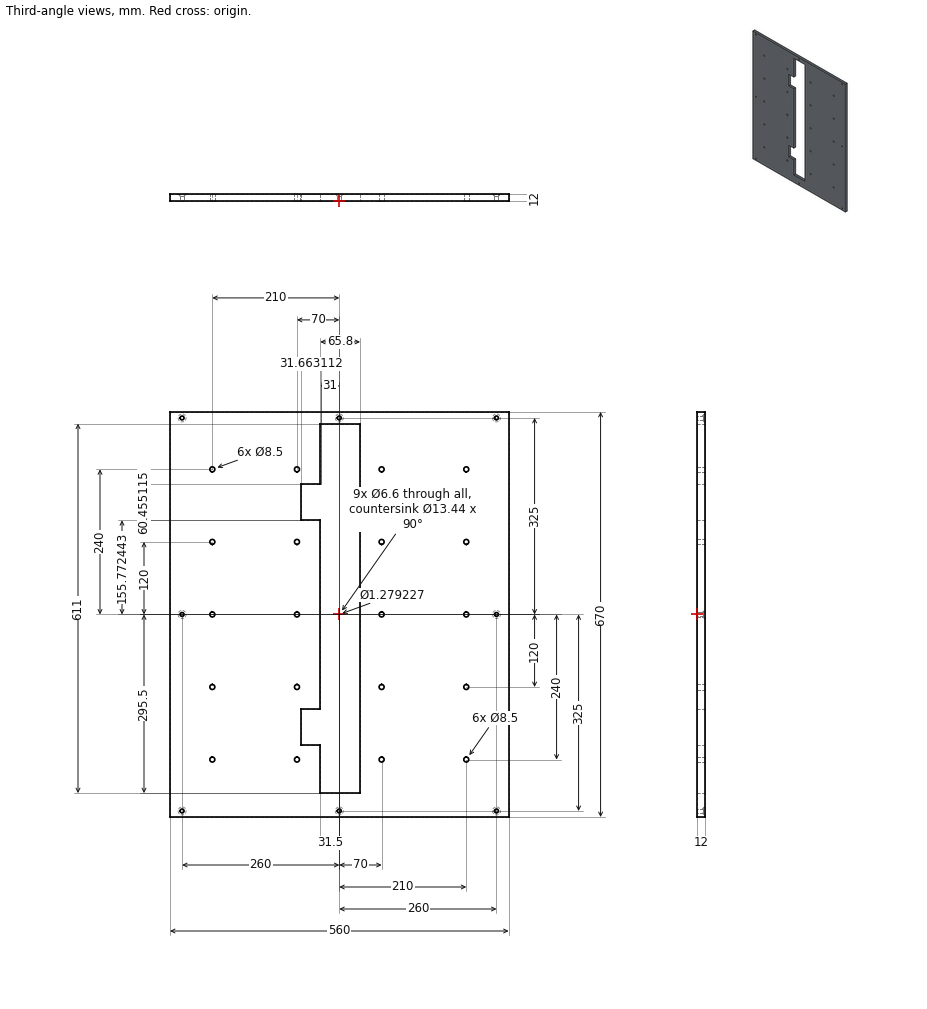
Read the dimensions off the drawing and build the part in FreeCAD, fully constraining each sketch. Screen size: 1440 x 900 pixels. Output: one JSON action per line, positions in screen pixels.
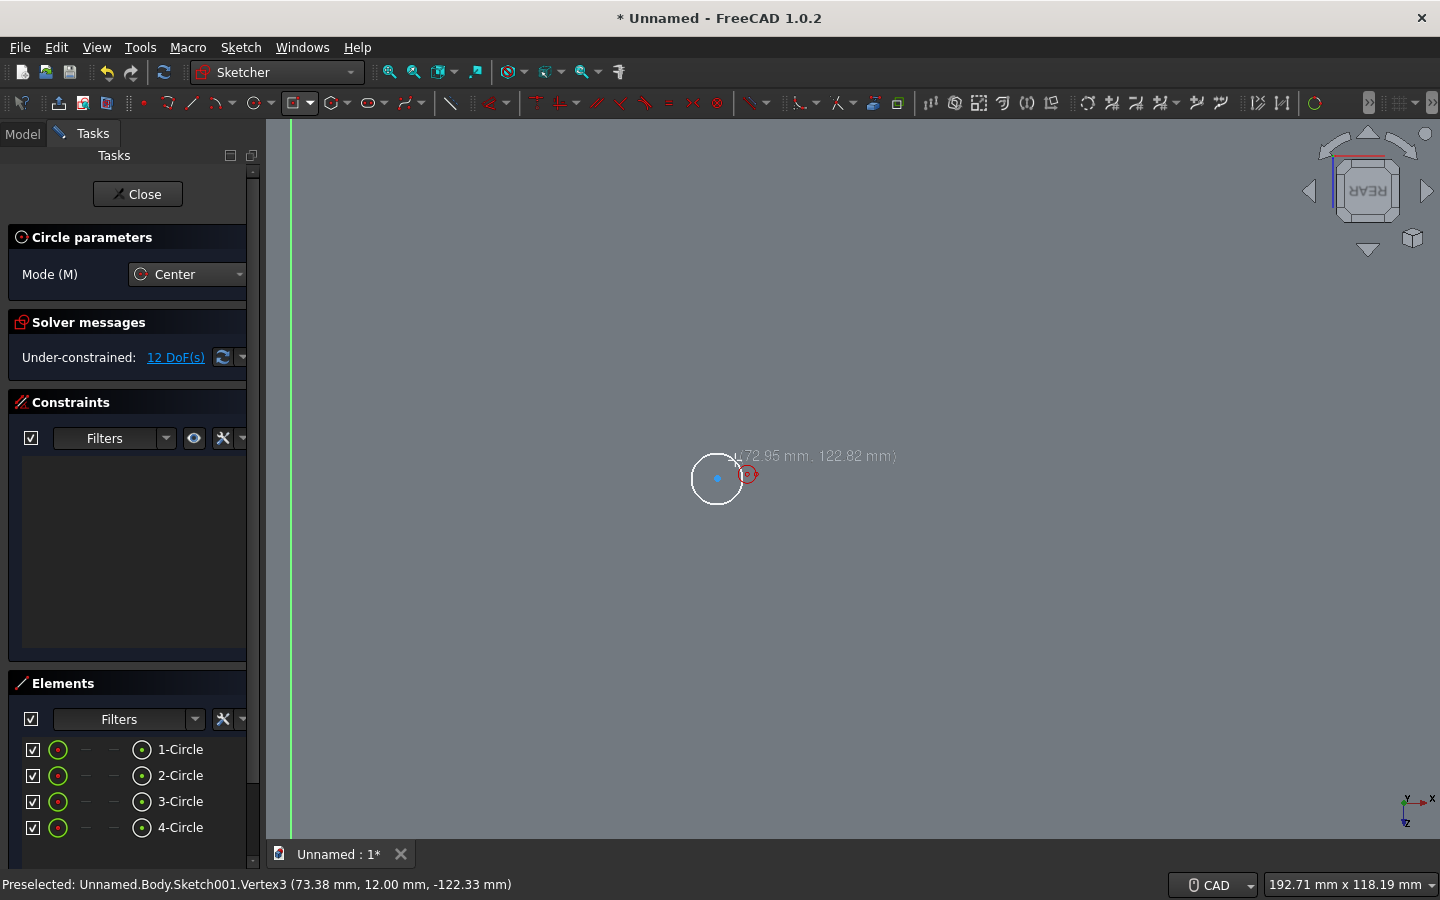
{"action": "scroll", "coordinate": [717, 479], "scroll_direction": "down", "scroll_amount": 6}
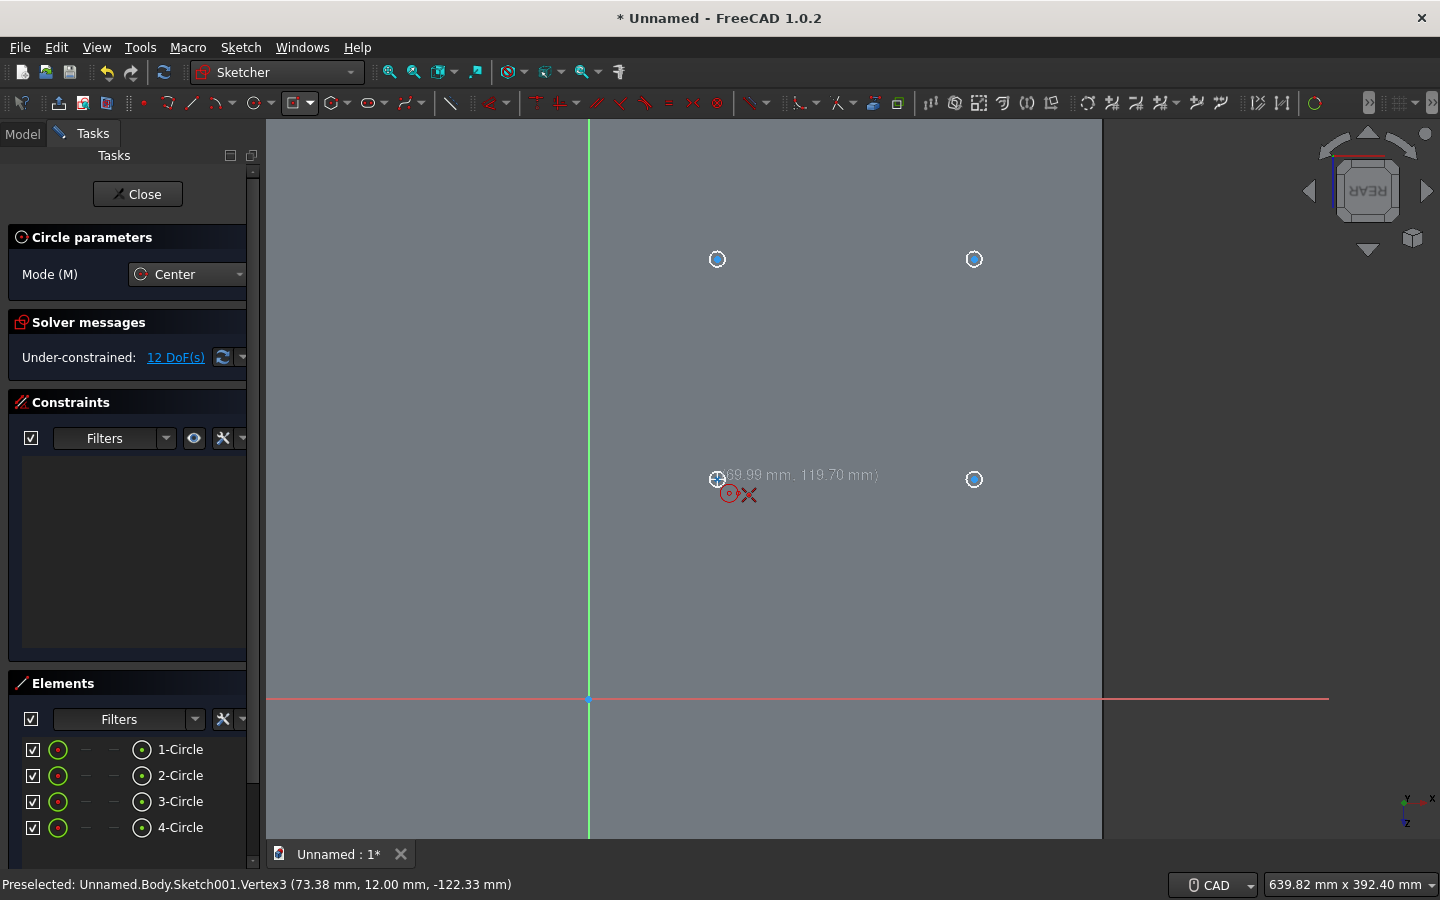
{"action": "scroll", "coordinate": [717, 699], "scroll_direction": "up", "scroll_amount": 6}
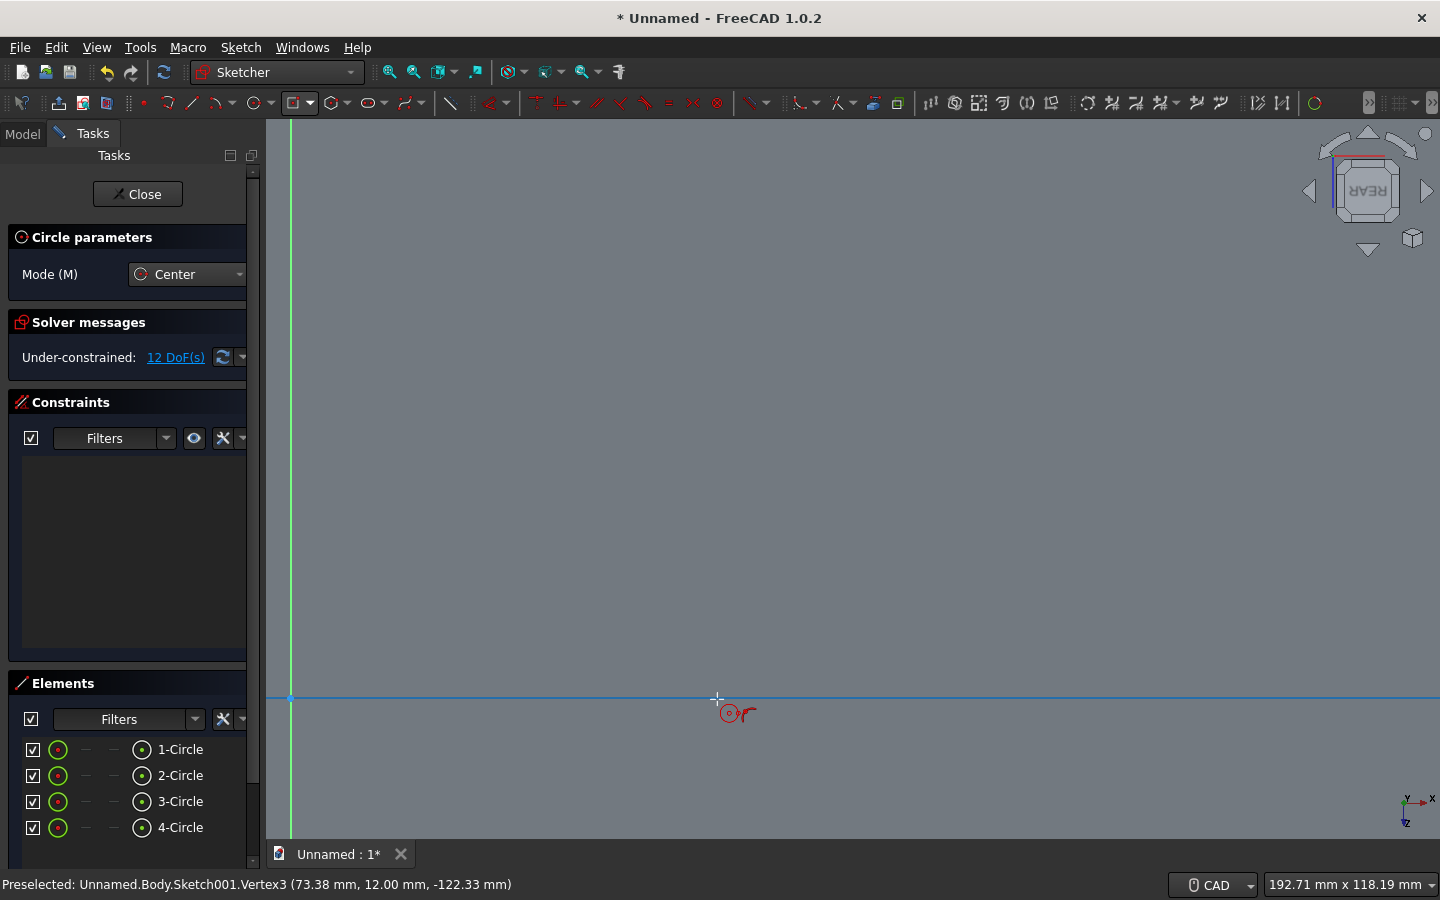
{"action": "left_click", "coordinate": [717, 698]}
{"action": "left_click", "coordinate": [735, 680]}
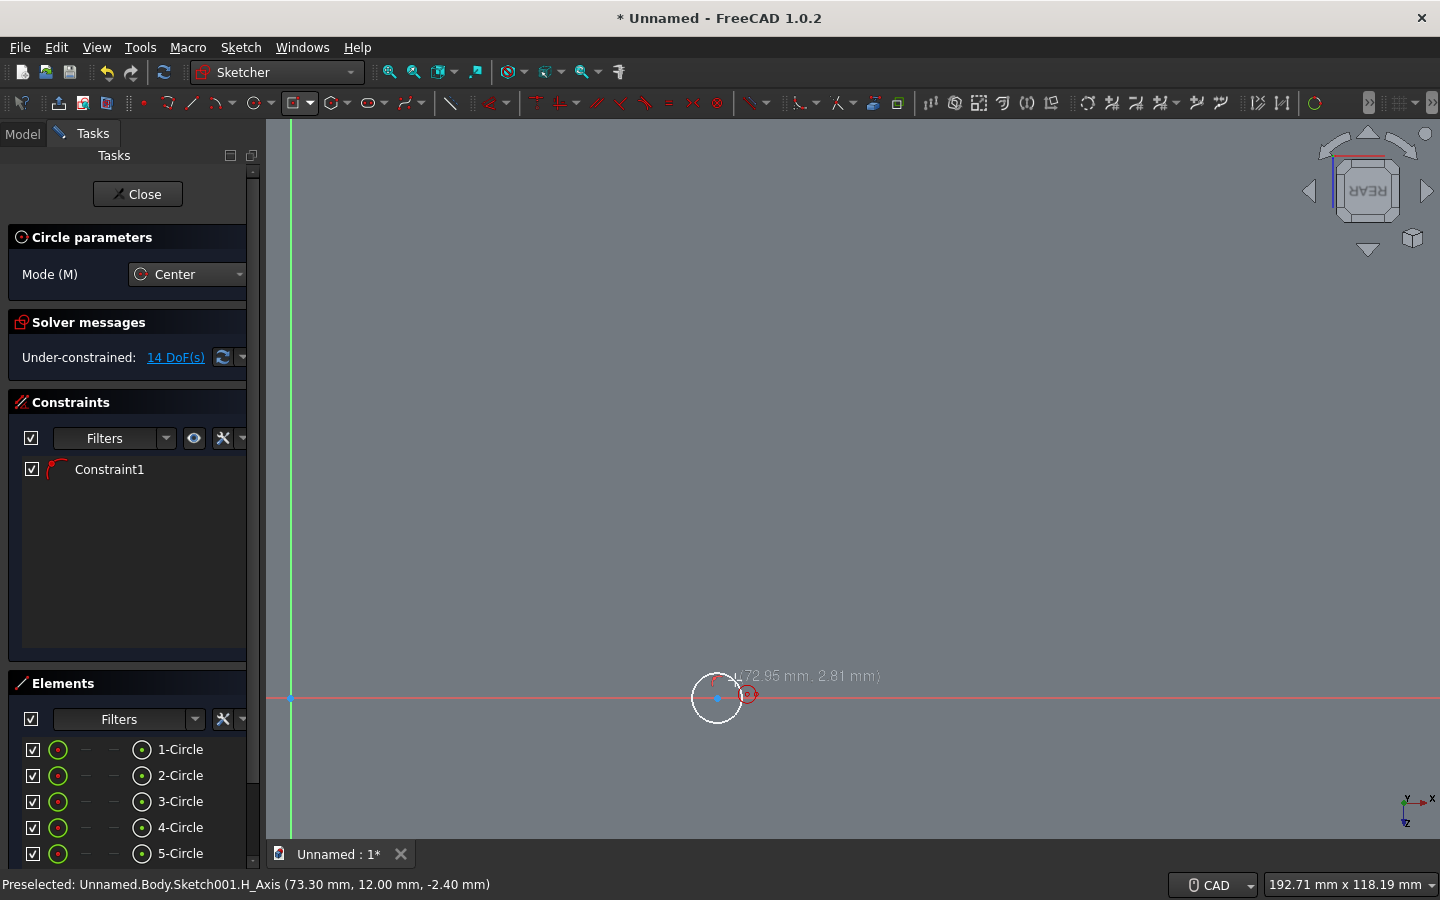
{"action": "scroll", "coordinate": [717, 700], "scroll_direction": "down", "scroll_amount": 6}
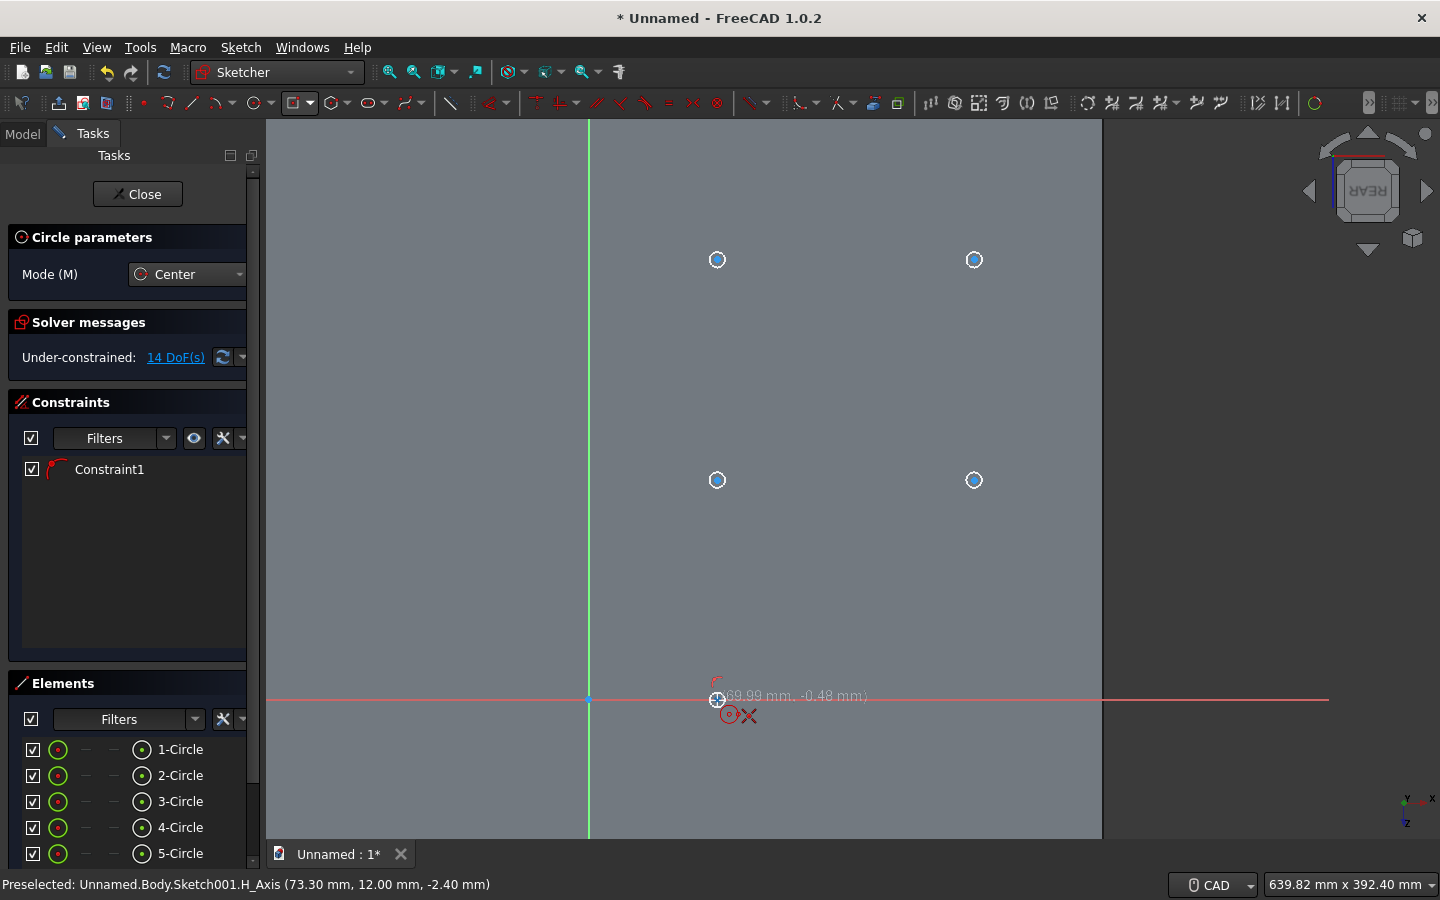
{"action": "scroll", "coordinate": [974, 700], "scroll_direction": "up", "scroll_amount": 6}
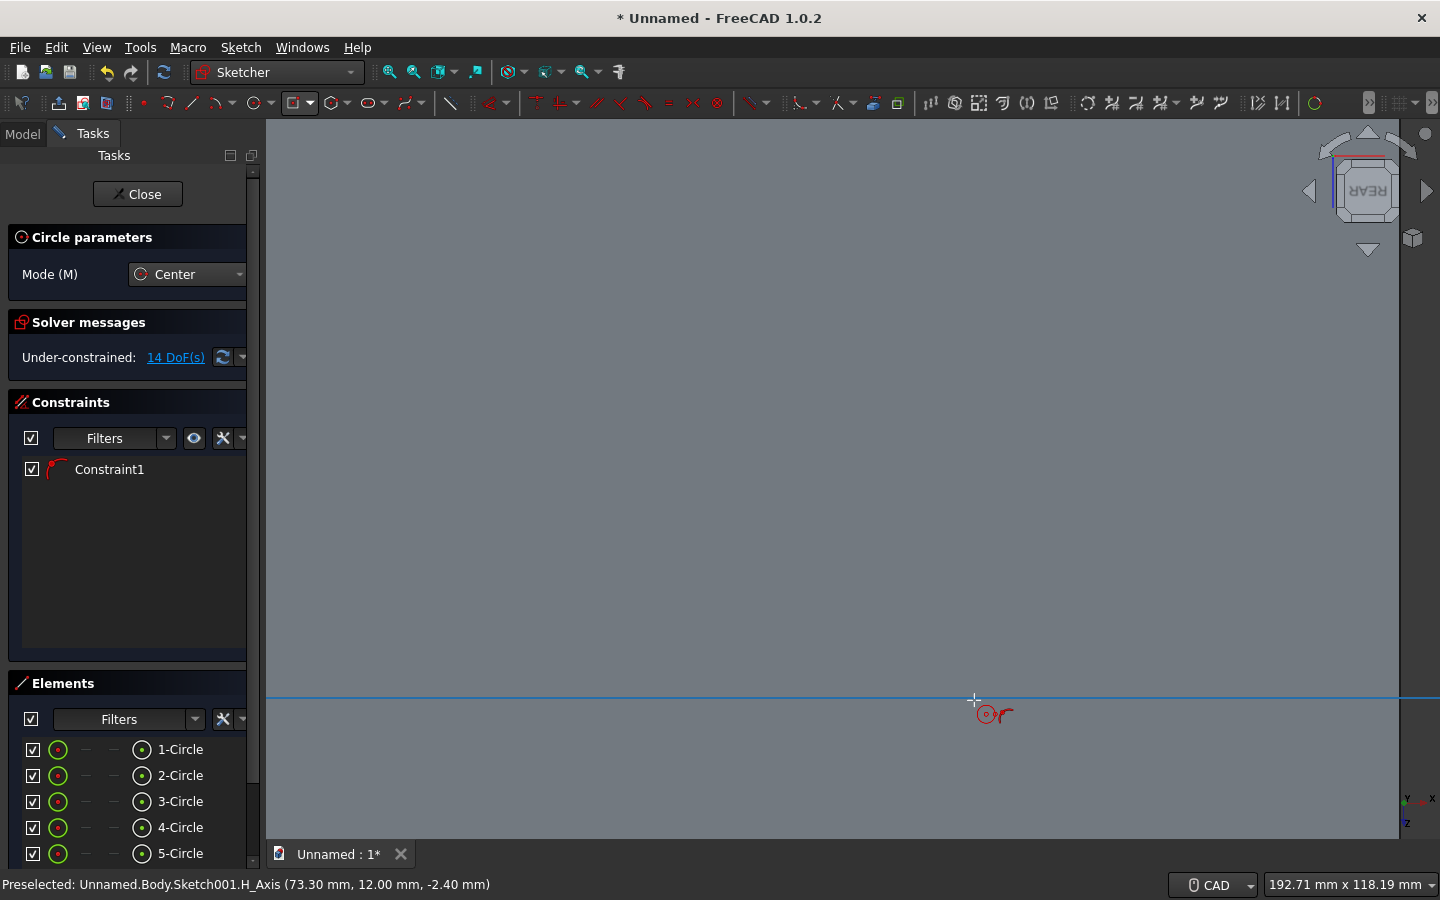
{"action": "left_click", "coordinate": [973, 698]}
{"action": "left_click", "coordinate": [991, 680]}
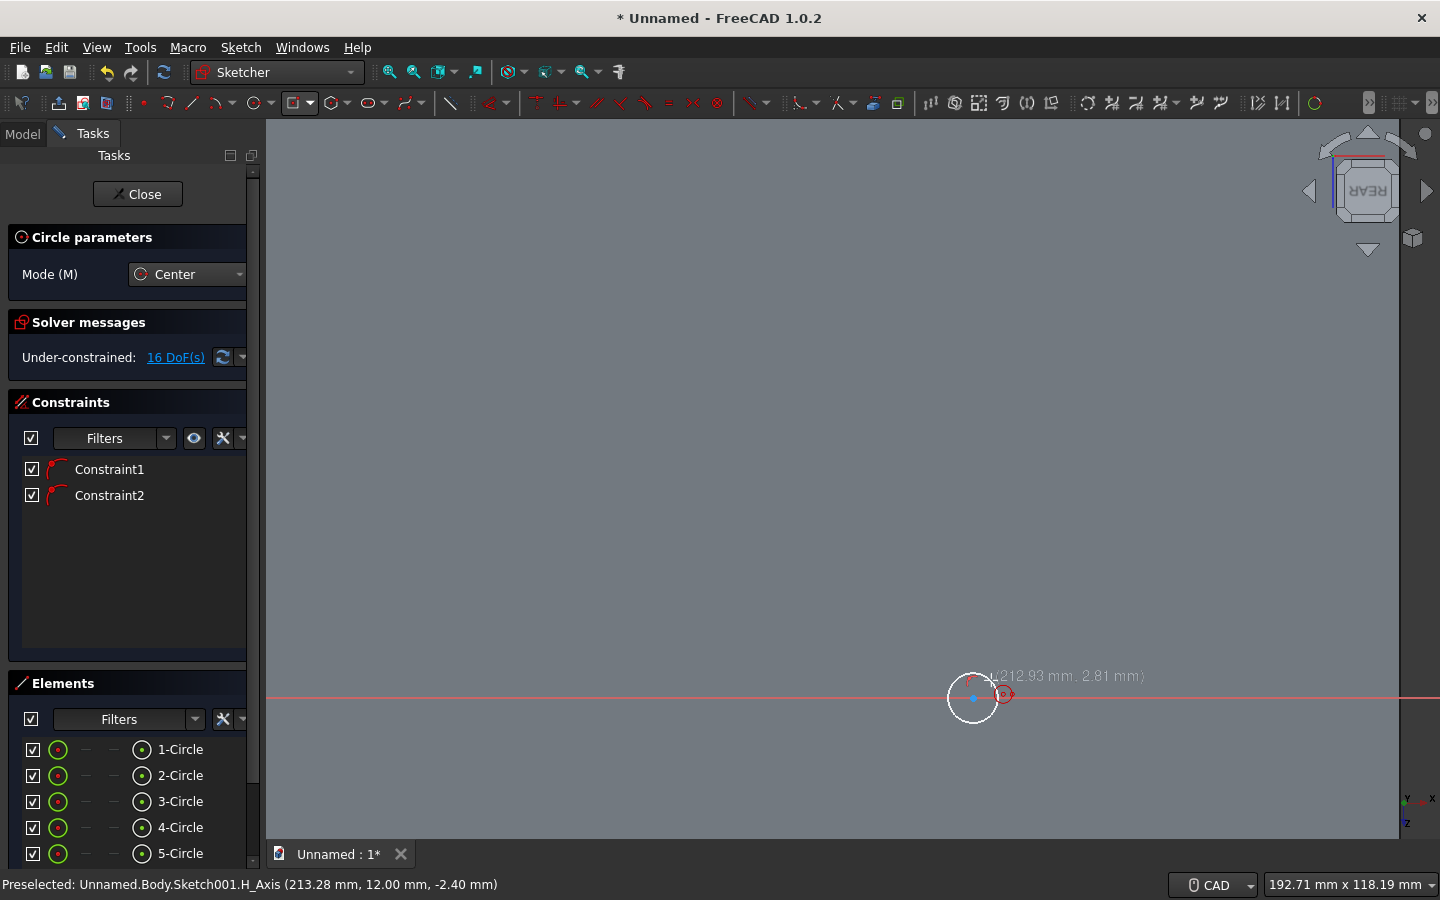
{"action": "scroll", "coordinate": [974, 700], "scroll_direction": "down", "scroll_amount": 6}